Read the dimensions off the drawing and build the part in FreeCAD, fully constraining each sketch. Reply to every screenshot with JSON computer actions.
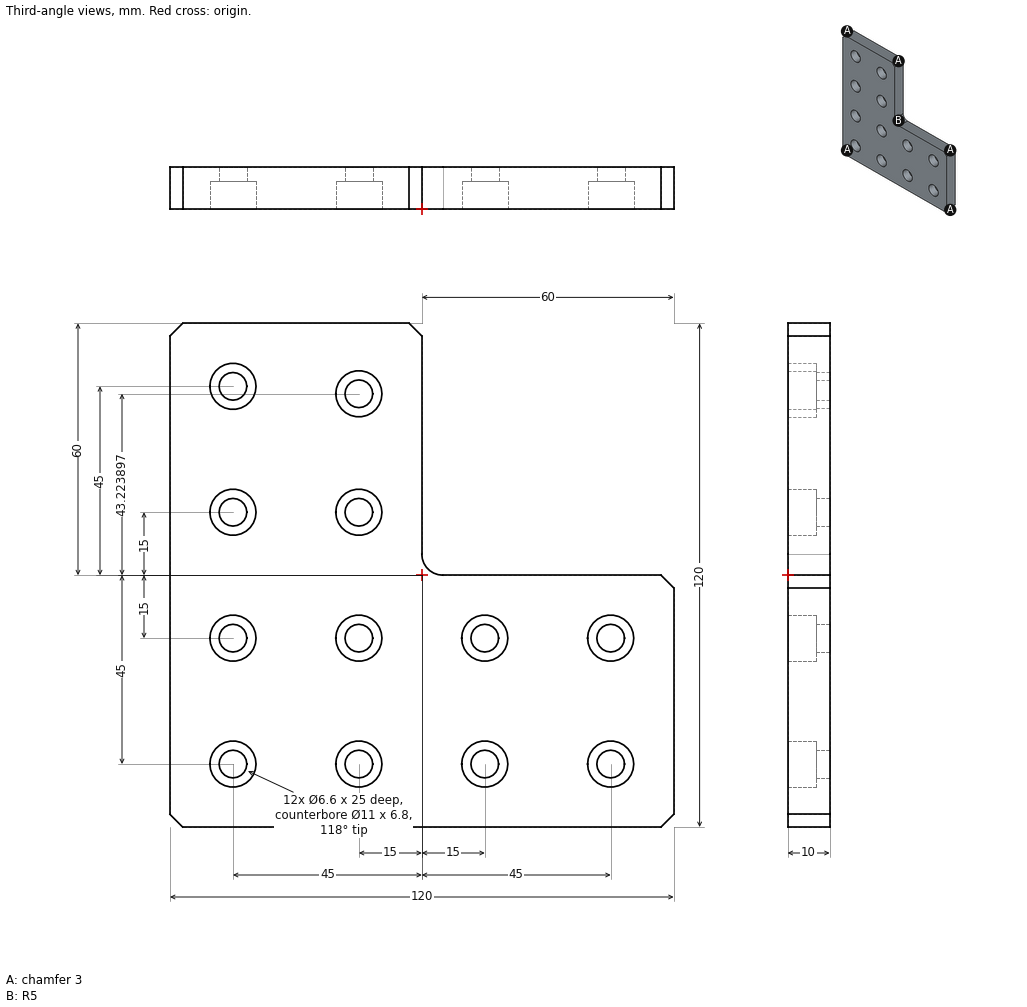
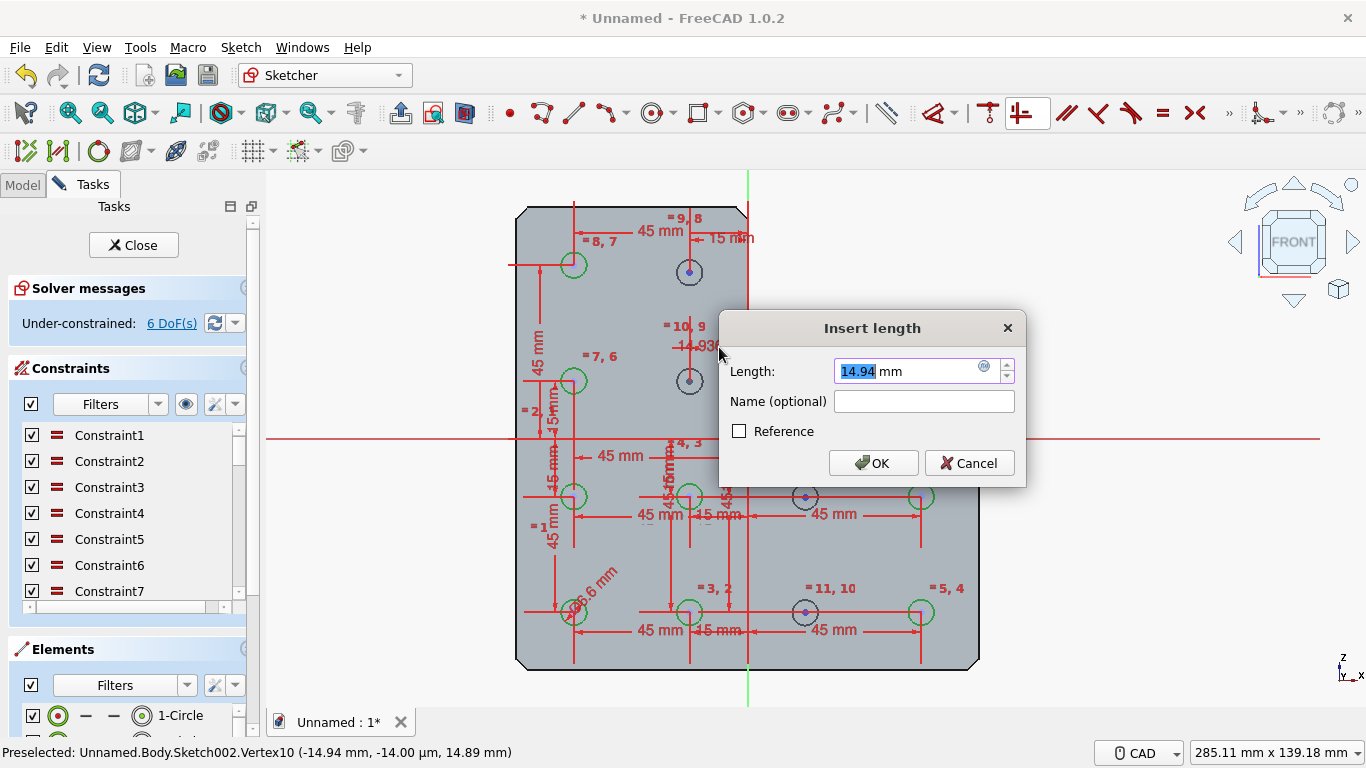
{"action": "type", "text": "15"}
{"action": "key", "text": "Return"}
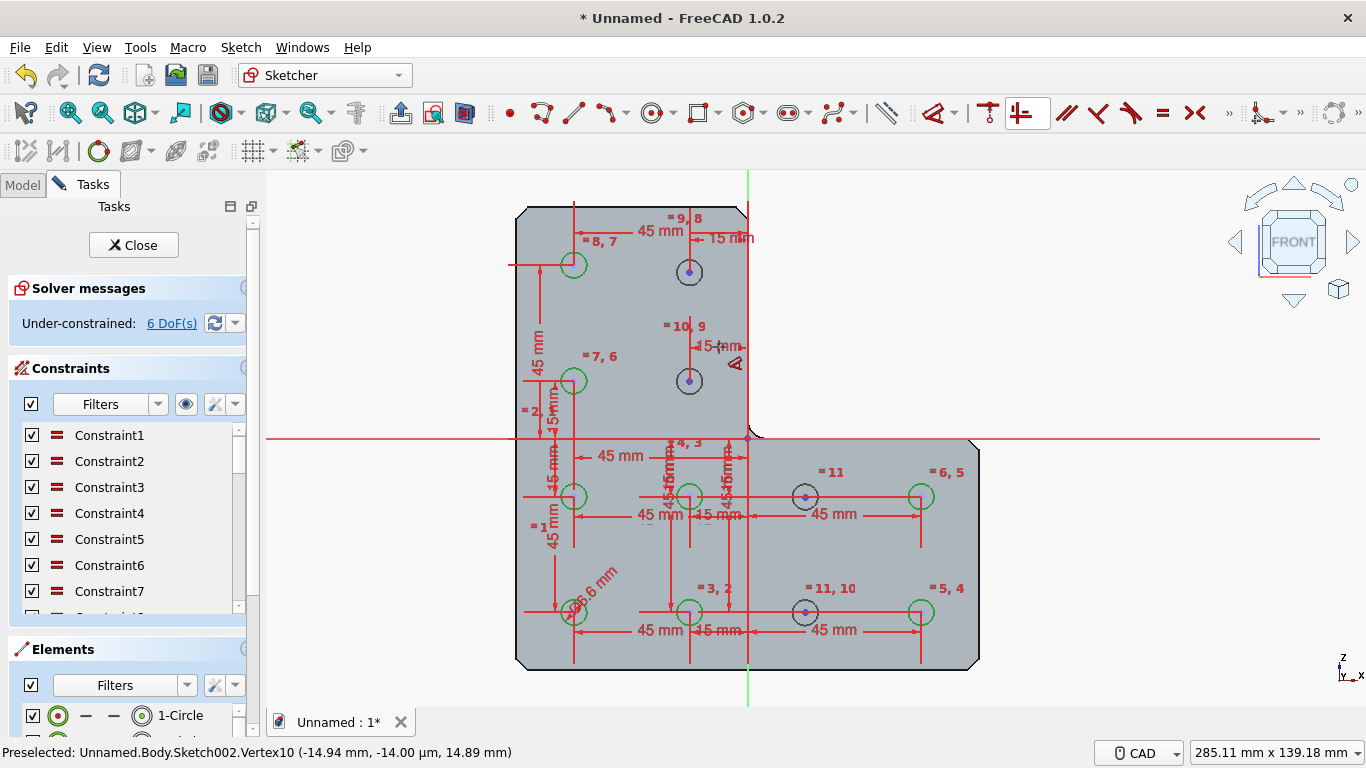
{"action": "left_click", "coordinate": [690, 381]}
{"action": "left_click", "coordinate": [656, 410]}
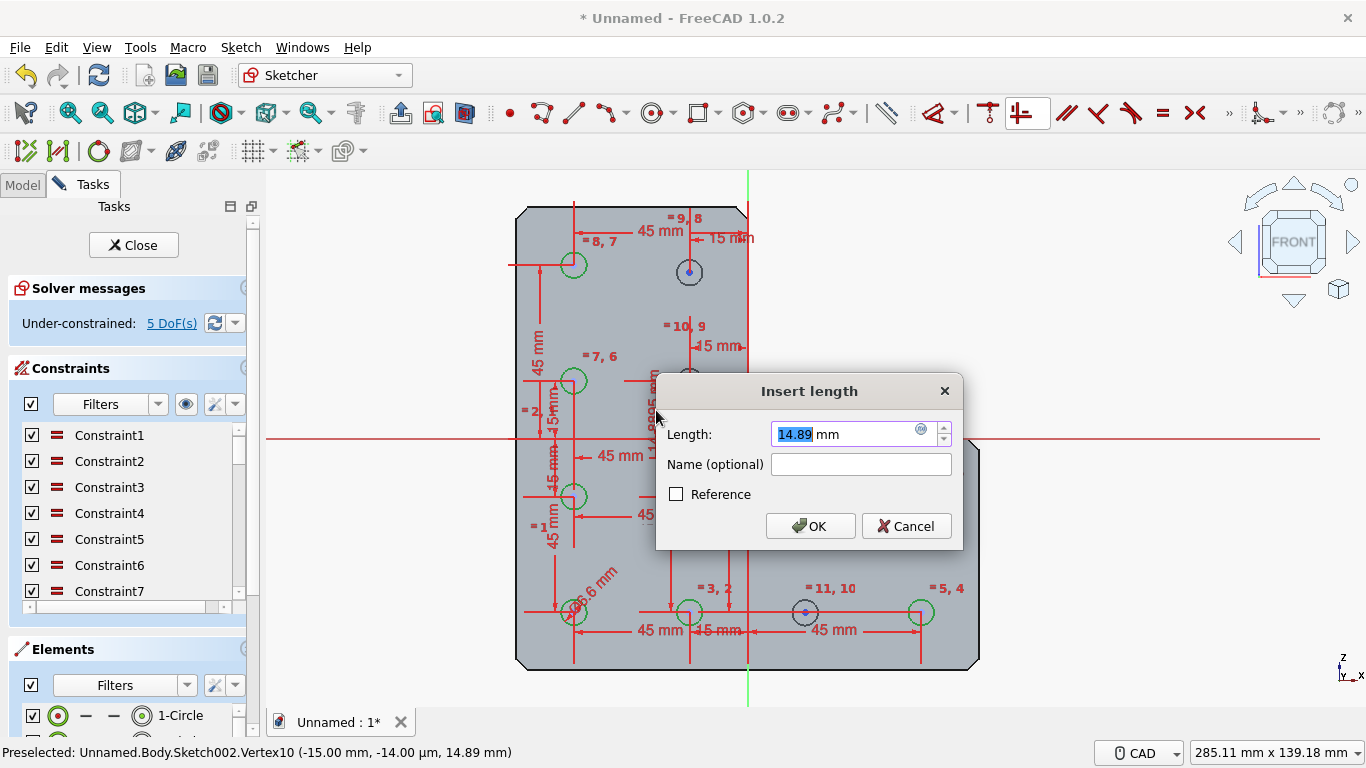
{"action": "type", "text": "15"}
{"action": "key", "text": "Return"}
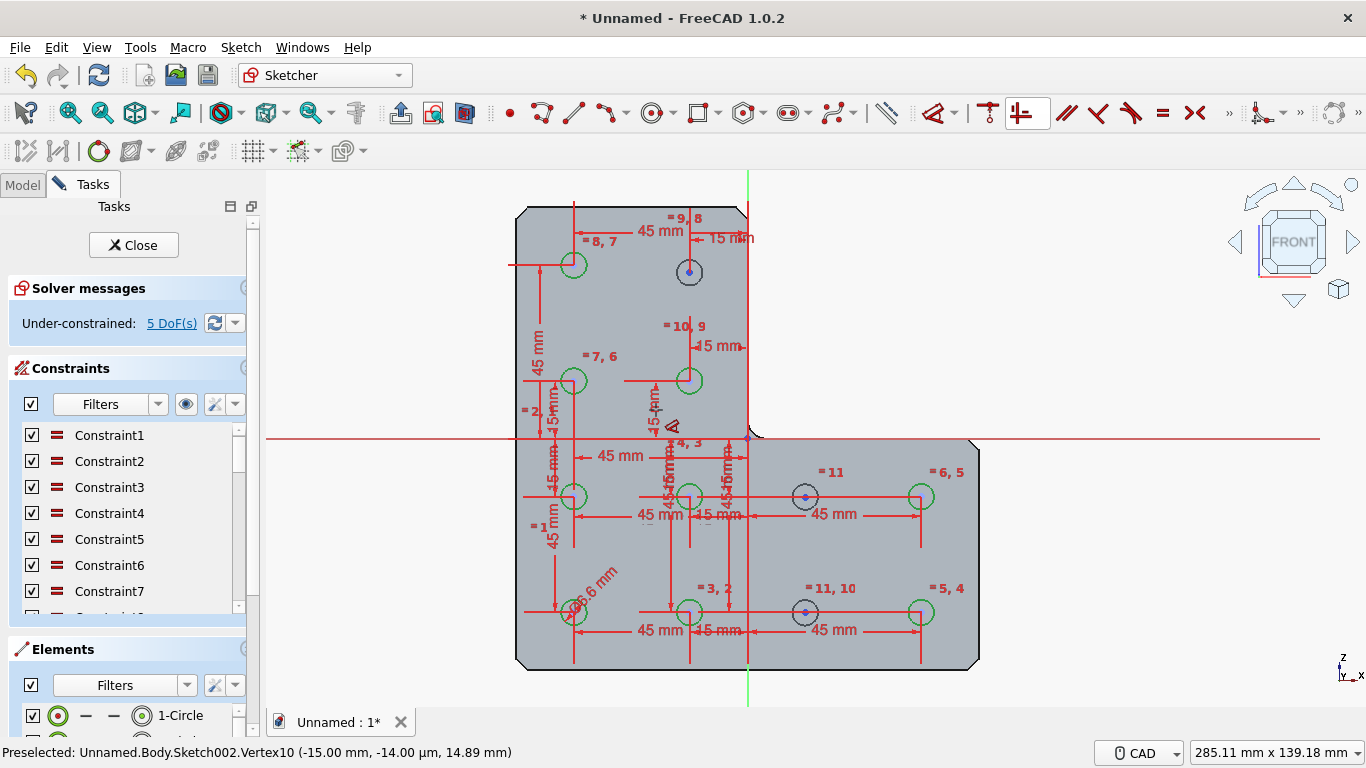
{"action": "left_click", "coordinate": [805, 613]}
{"action": "left_click", "coordinate": [776, 405]}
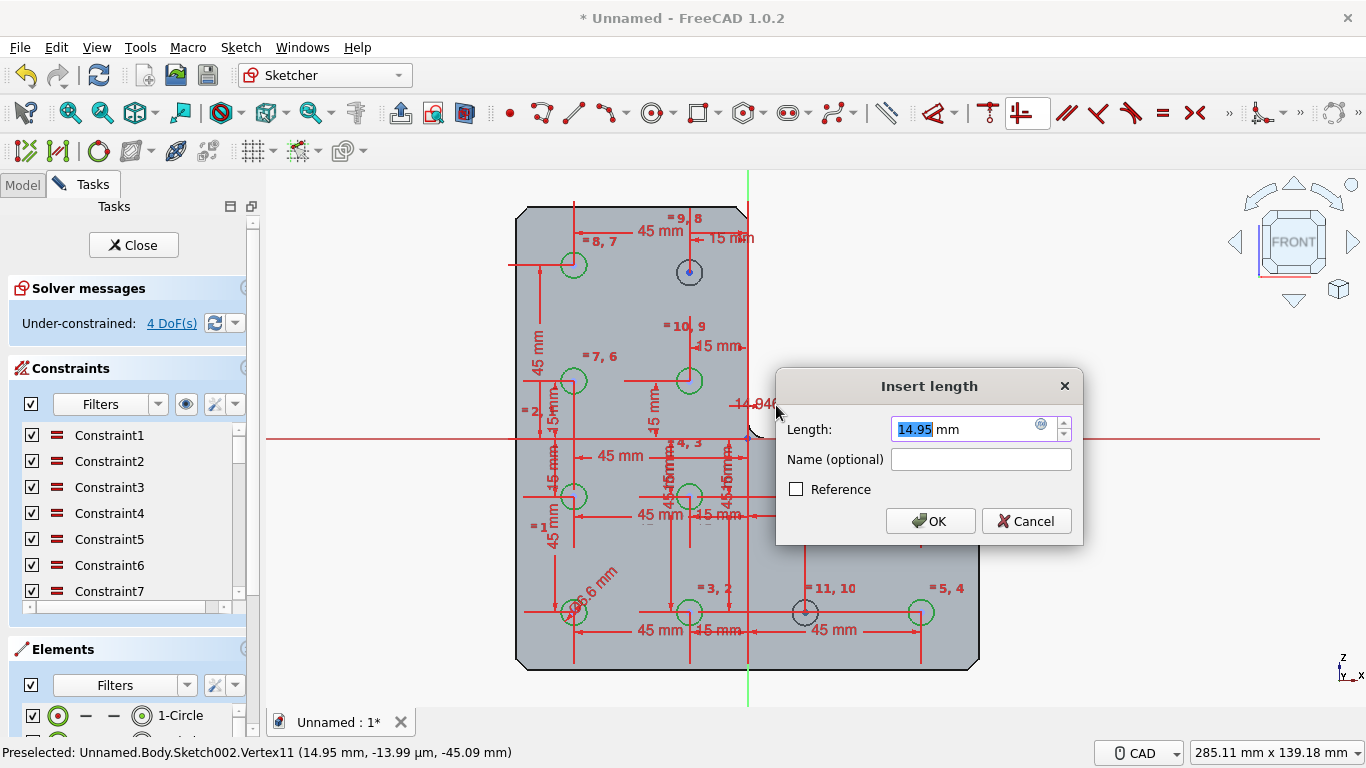
{"action": "type", "text": "15"}
{"action": "key", "text": "Return"}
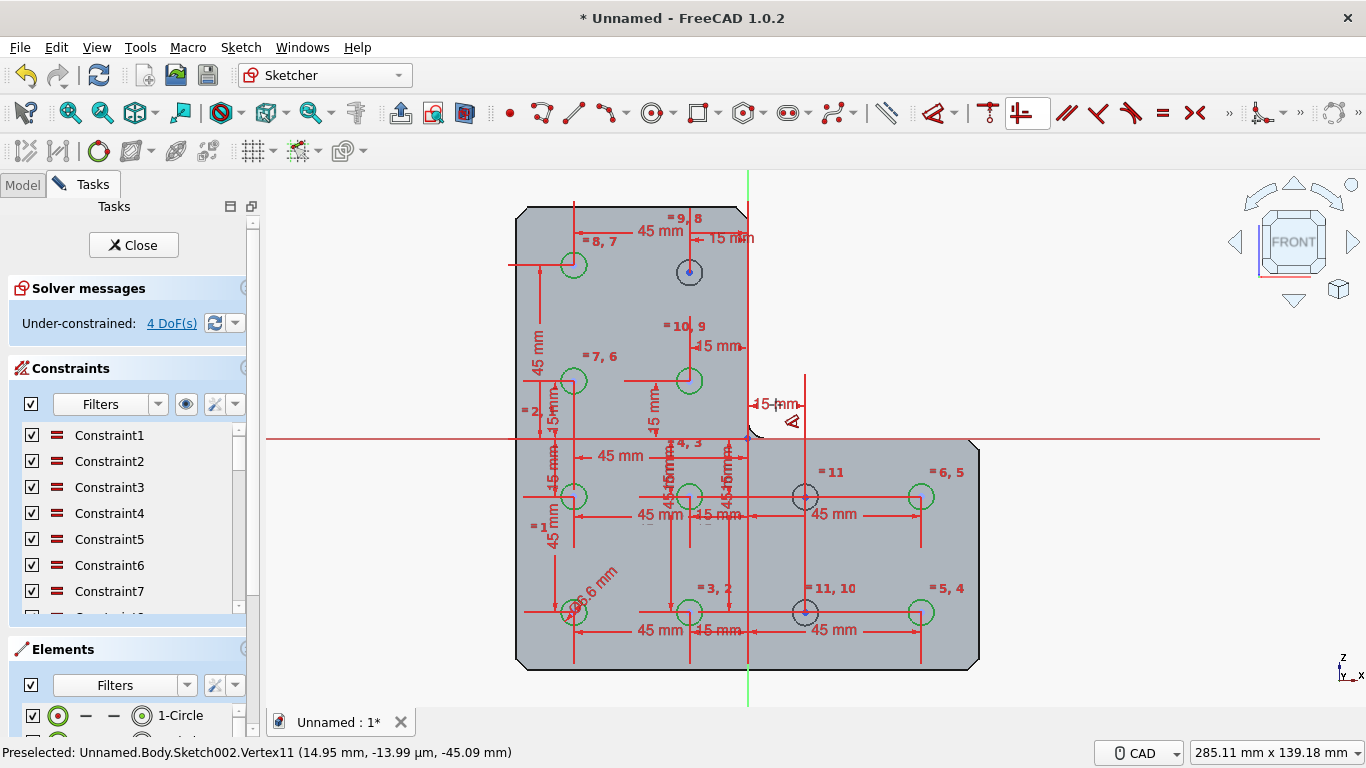
{"action": "left_click", "coordinate": [805, 613]}
{"action": "left_click", "coordinate": [839, 486]}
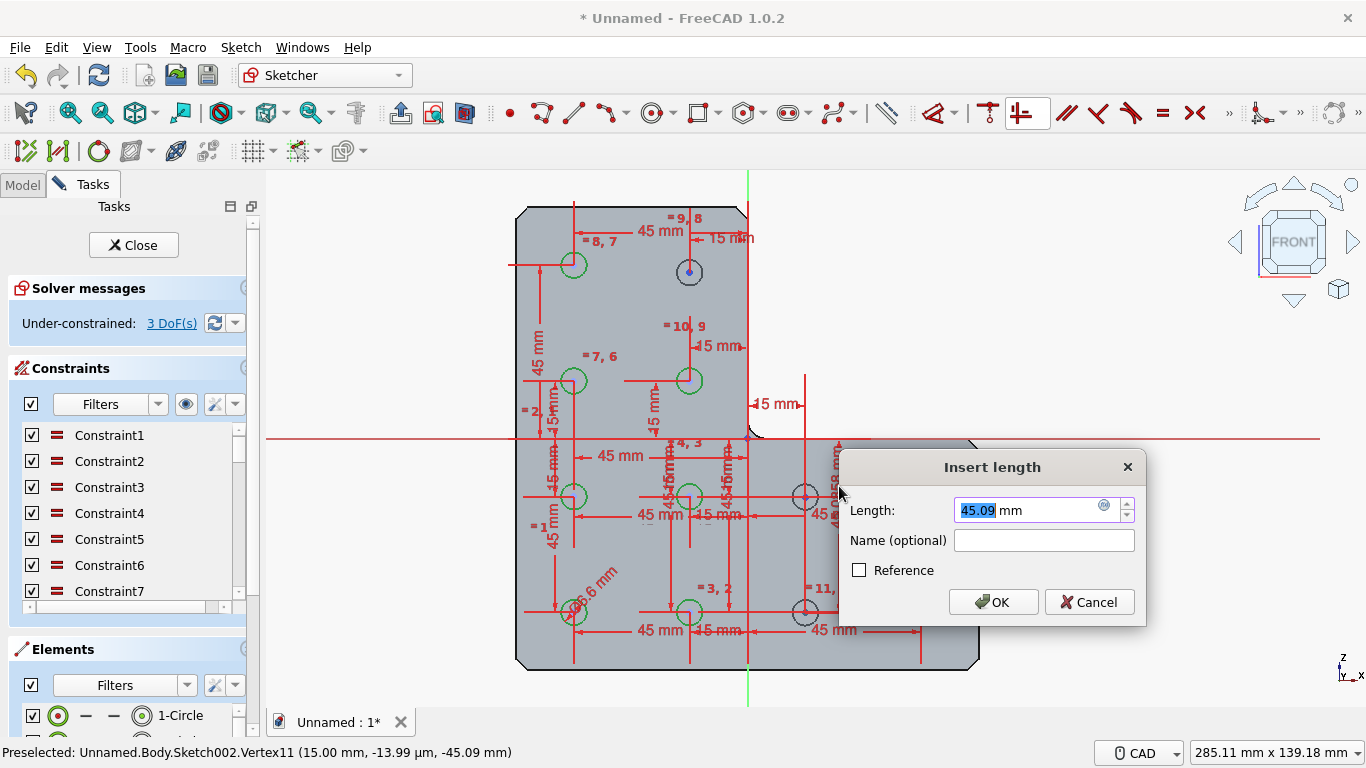
{"action": "type", "text": "45"}
{"action": "key", "text": "Return"}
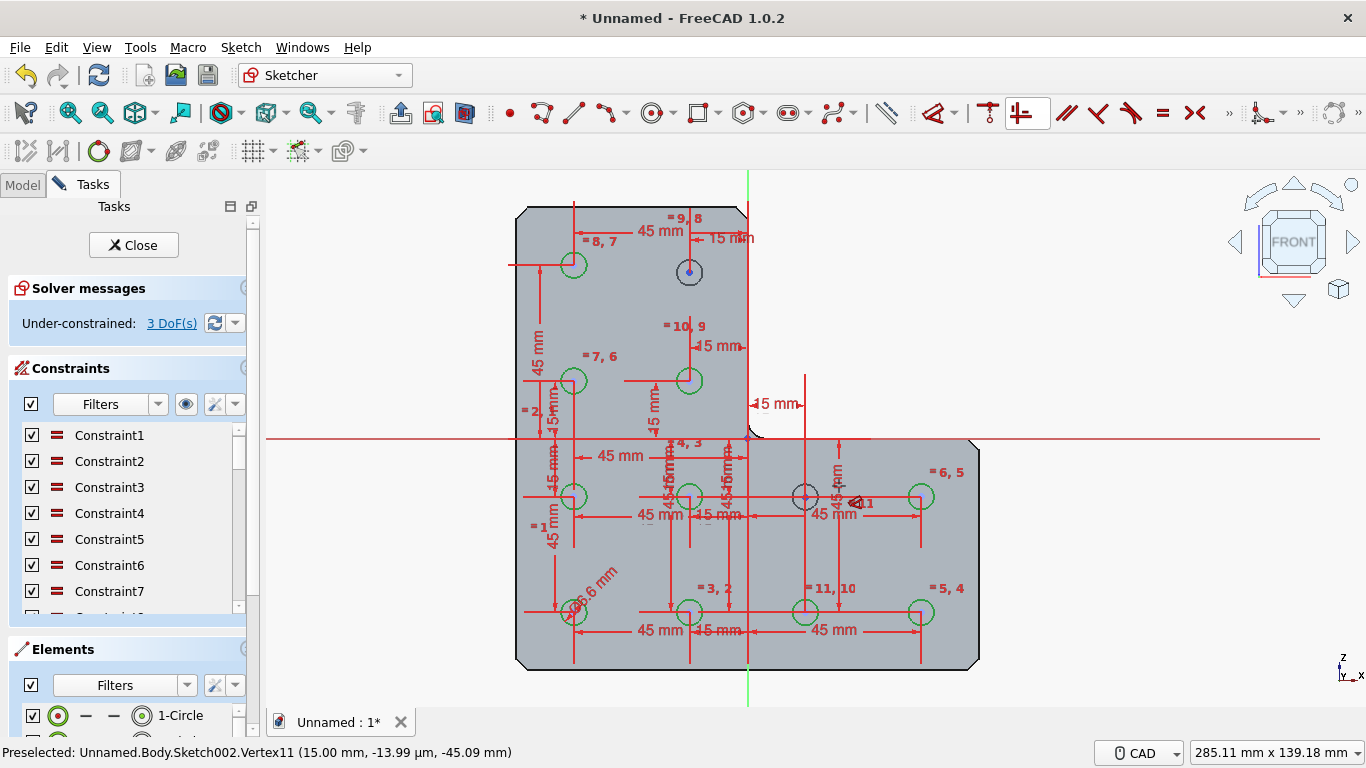
{"action": "left_click", "coordinate": [805, 497]}
{"action": "left_click", "coordinate": [776, 555]}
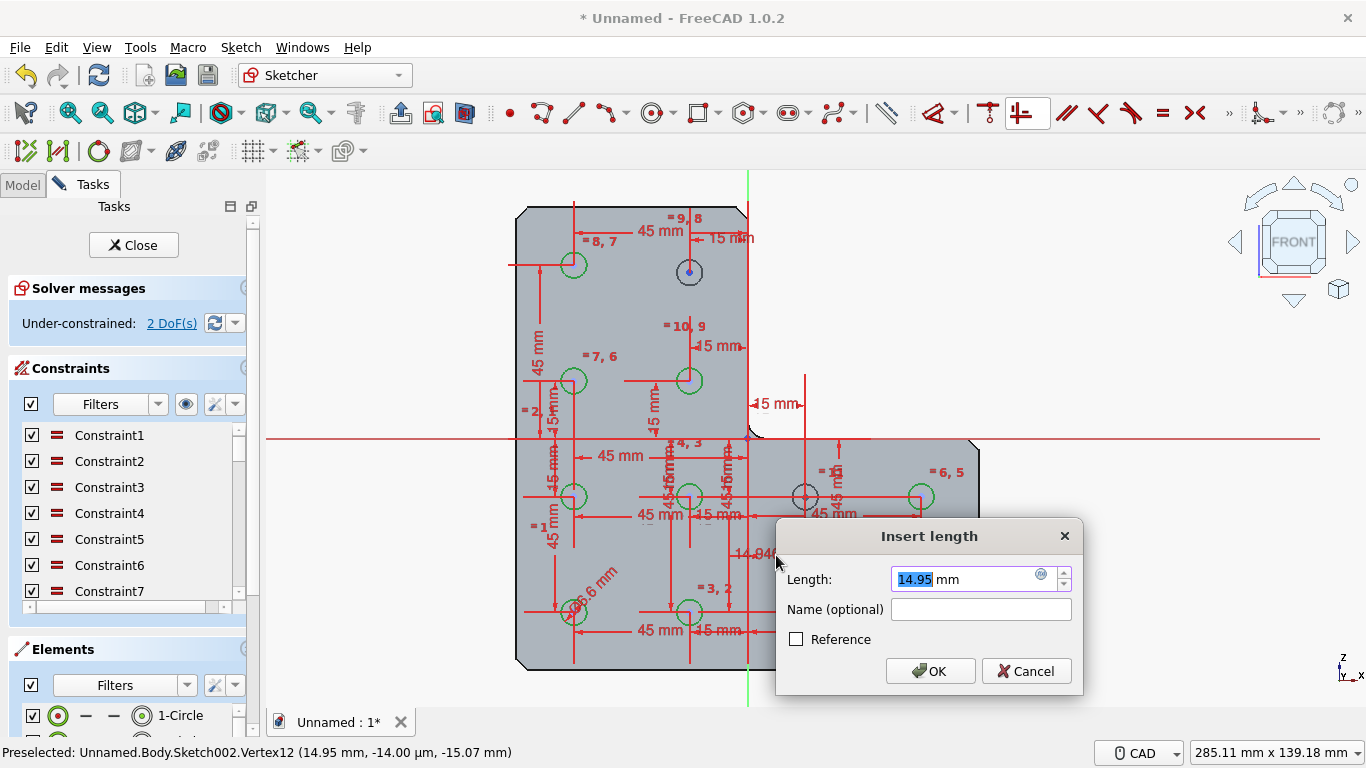
{"action": "type", "text": "15"}
{"action": "key", "text": "Return"}